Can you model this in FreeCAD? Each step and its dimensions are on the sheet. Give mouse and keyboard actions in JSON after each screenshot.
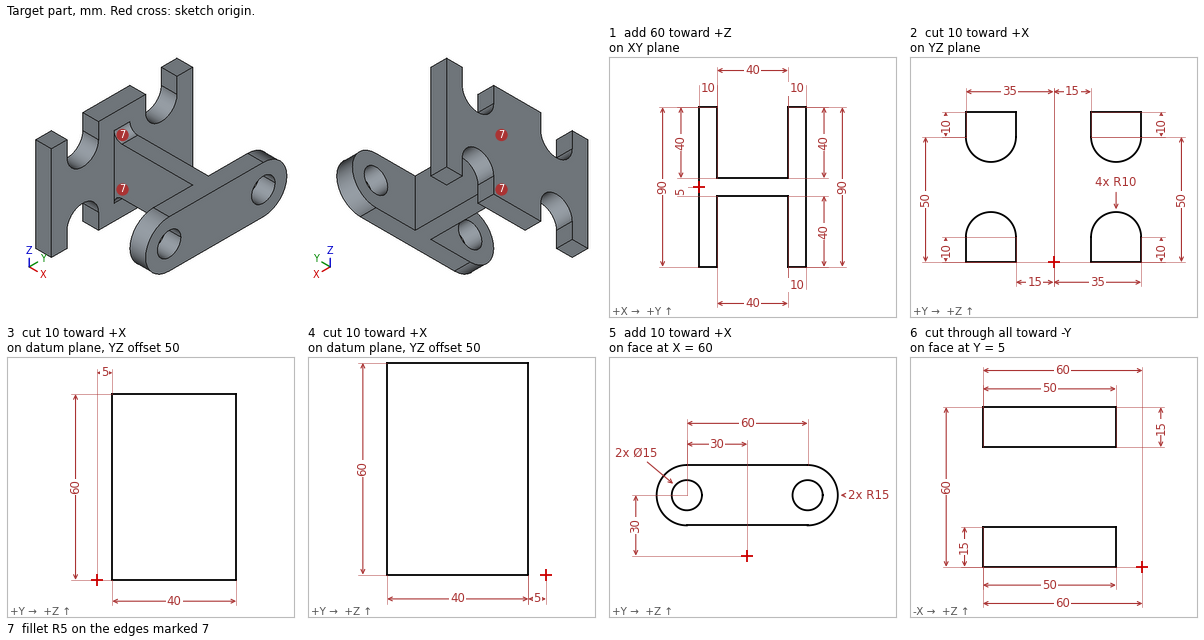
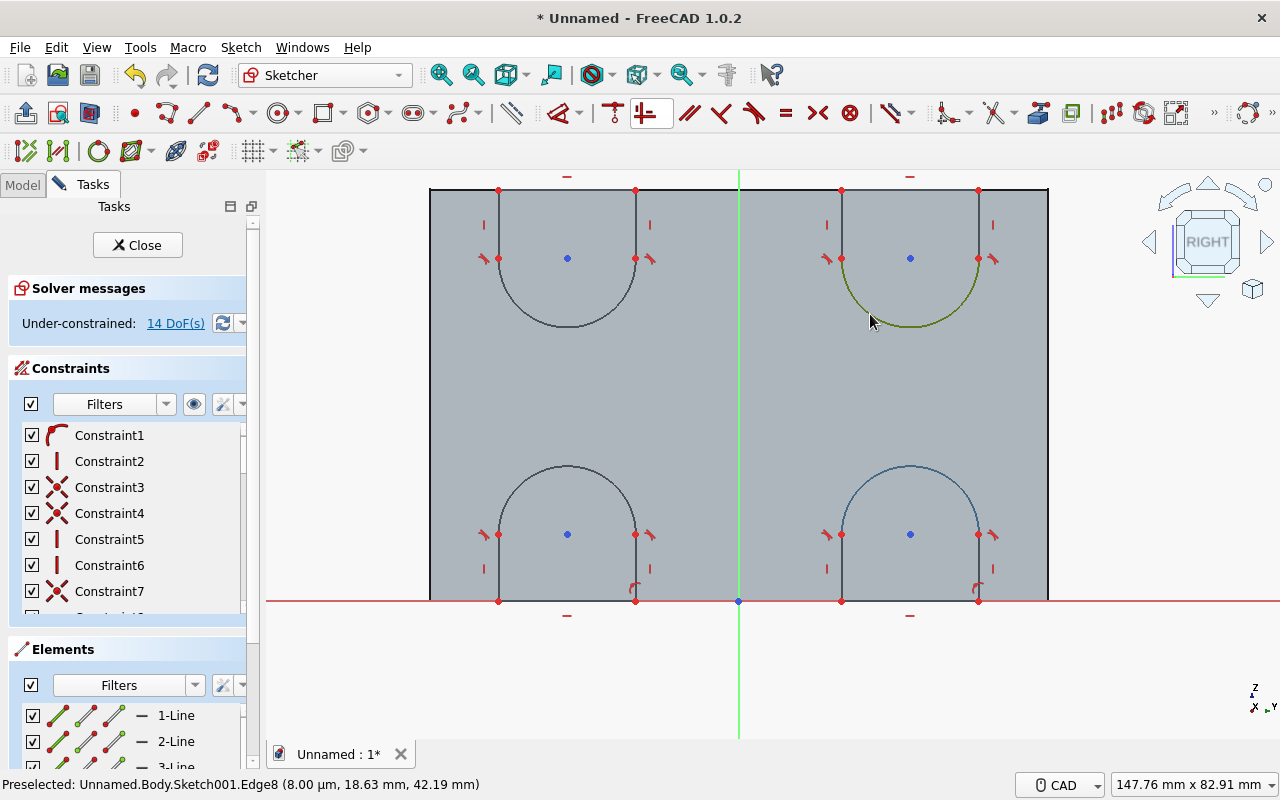
{"action": "left_click", "coordinate": [608, 479]}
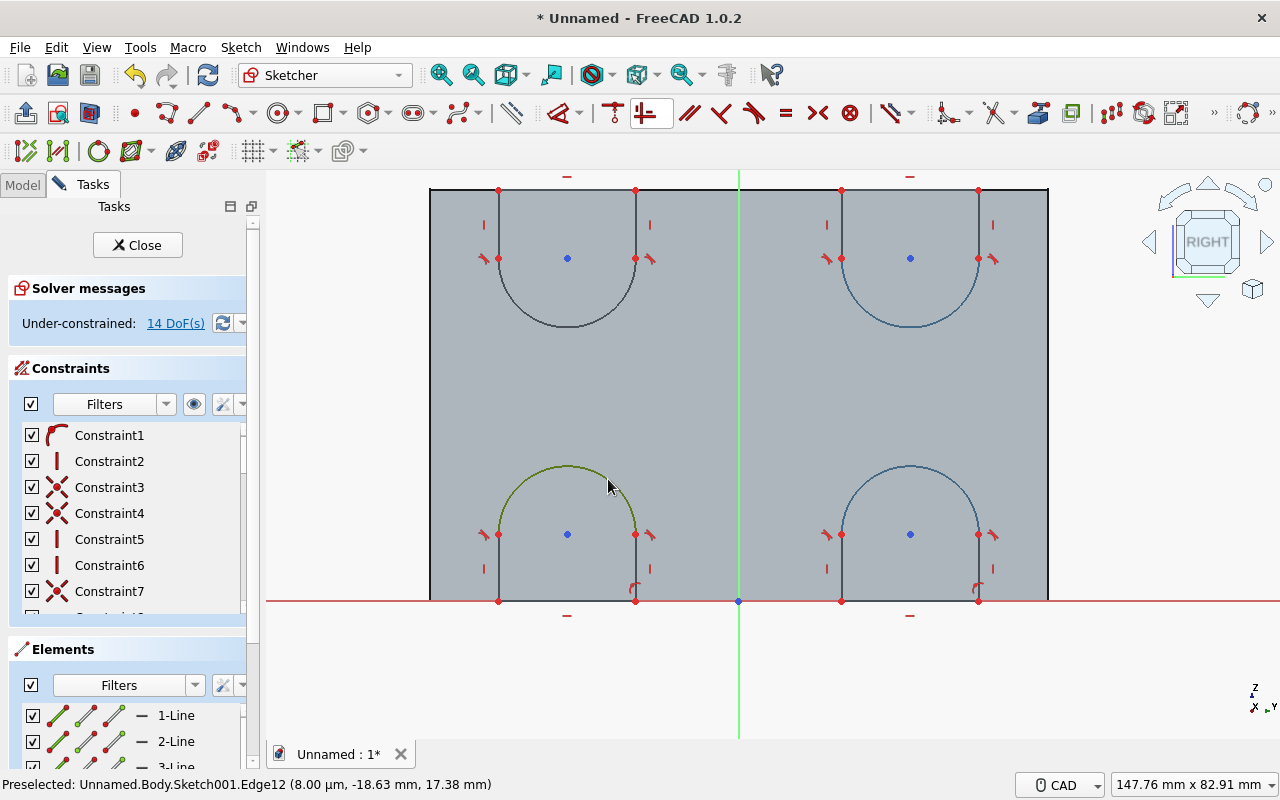
{"action": "left_click", "coordinate": [527, 314]}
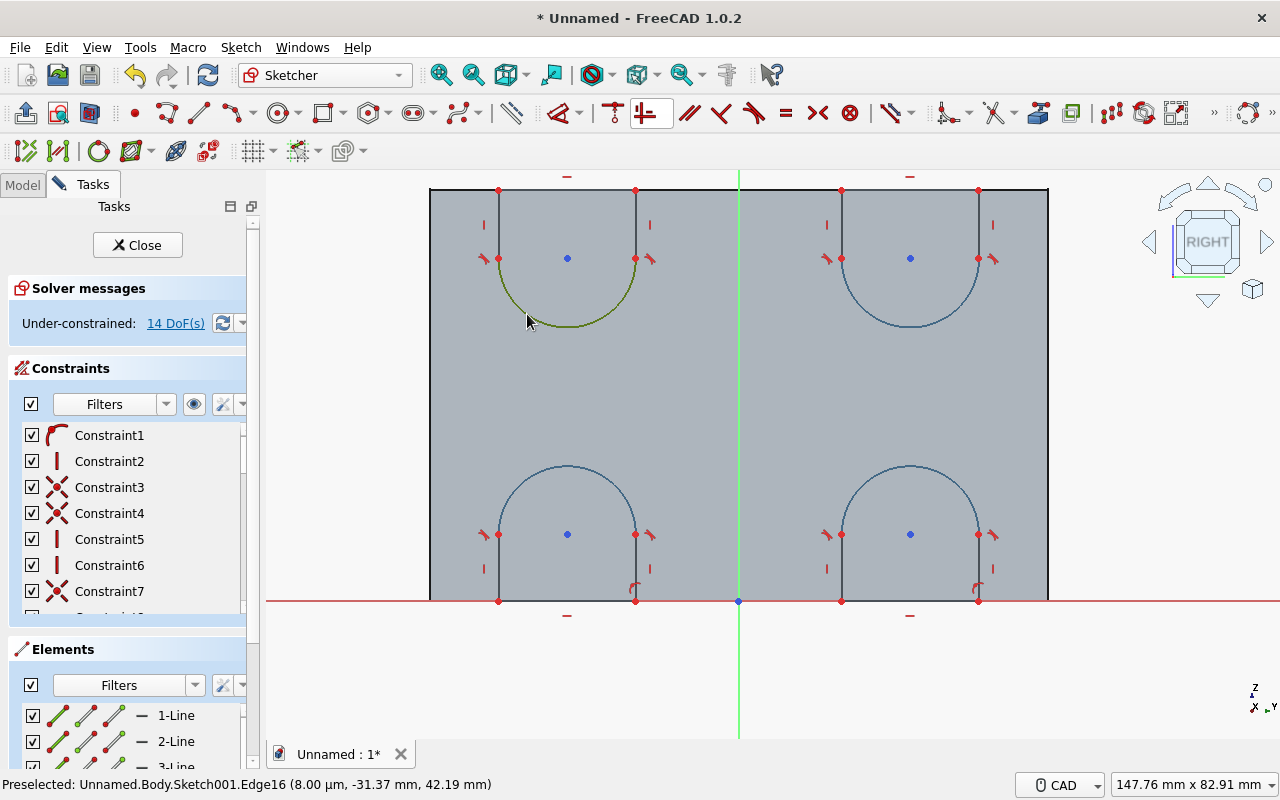
{"action": "left_click", "coordinate": [786, 114]}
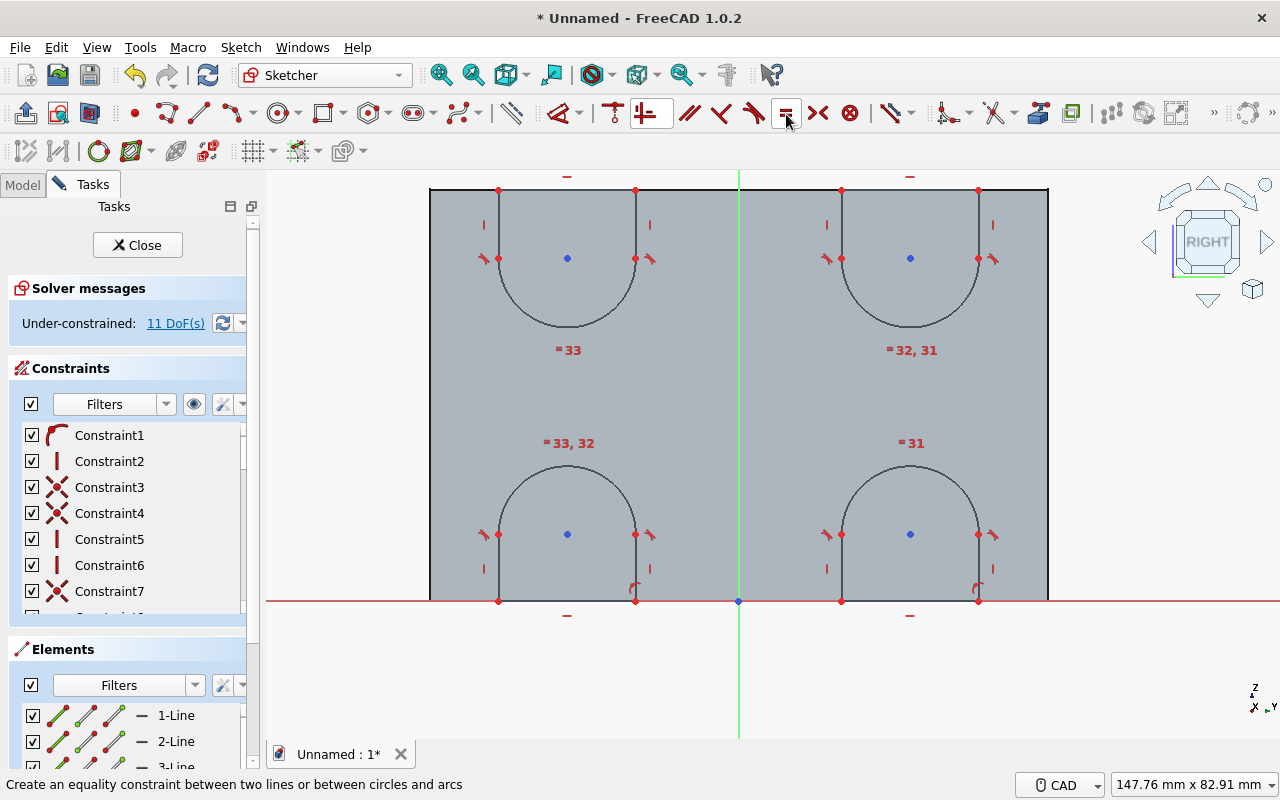
{"action": "left_click", "coordinate": [558, 114]}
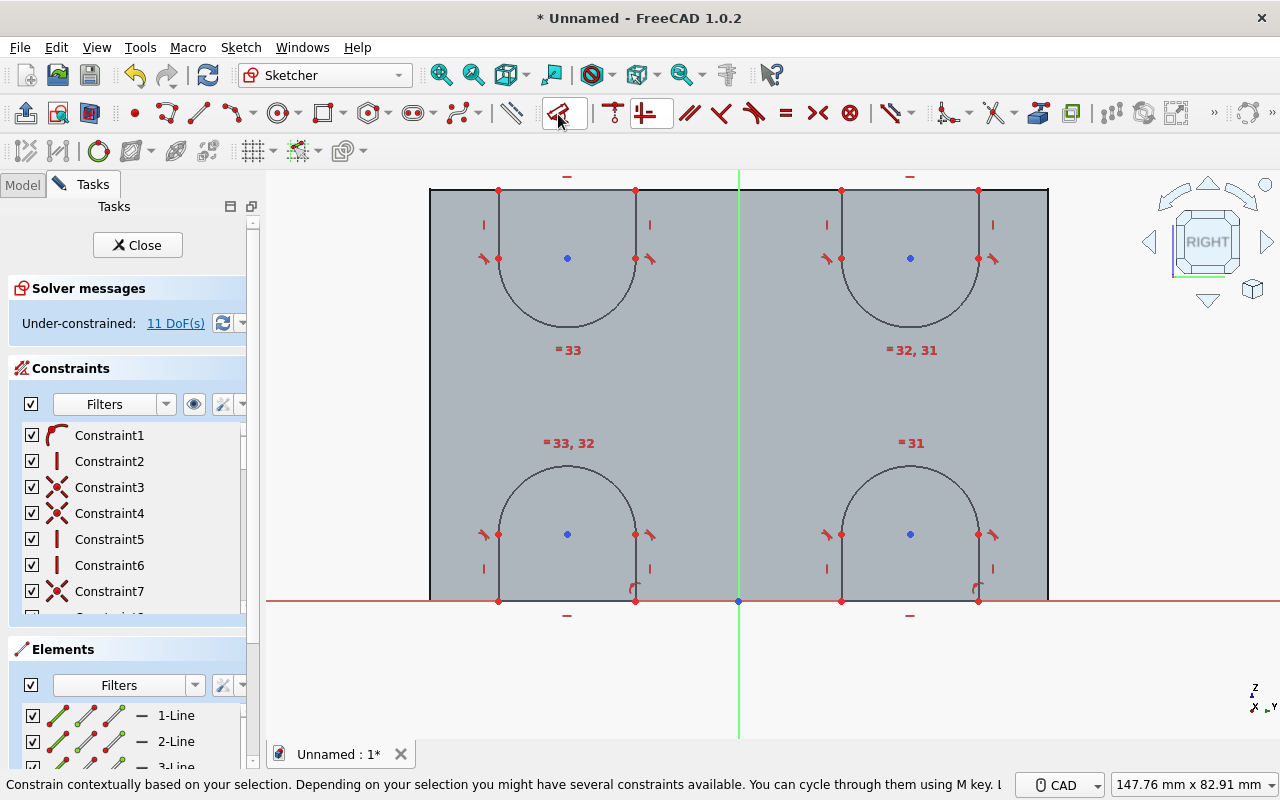
{"action": "left_click", "coordinate": [951, 479]}
{"action": "left_click", "coordinate": [970, 453]}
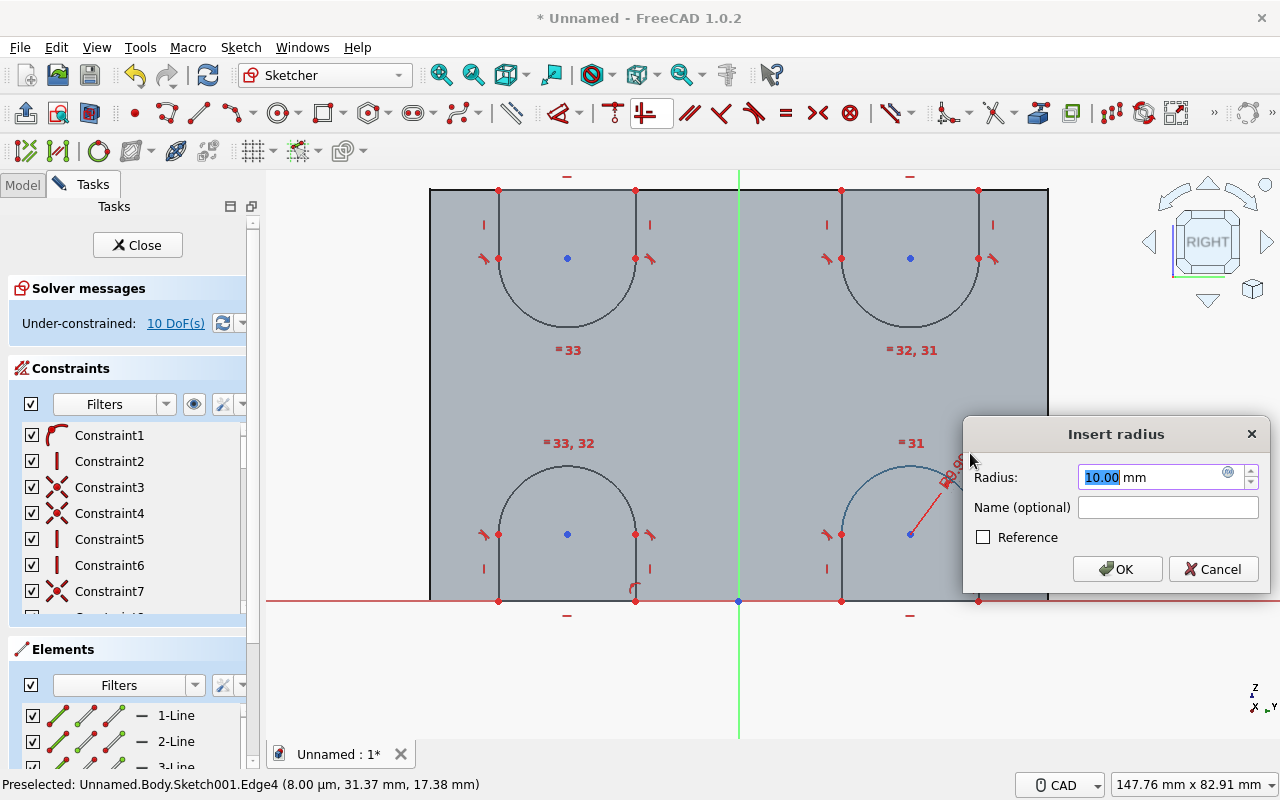
{"action": "type", "text": "10"}
{"action": "key", "text": "Return"}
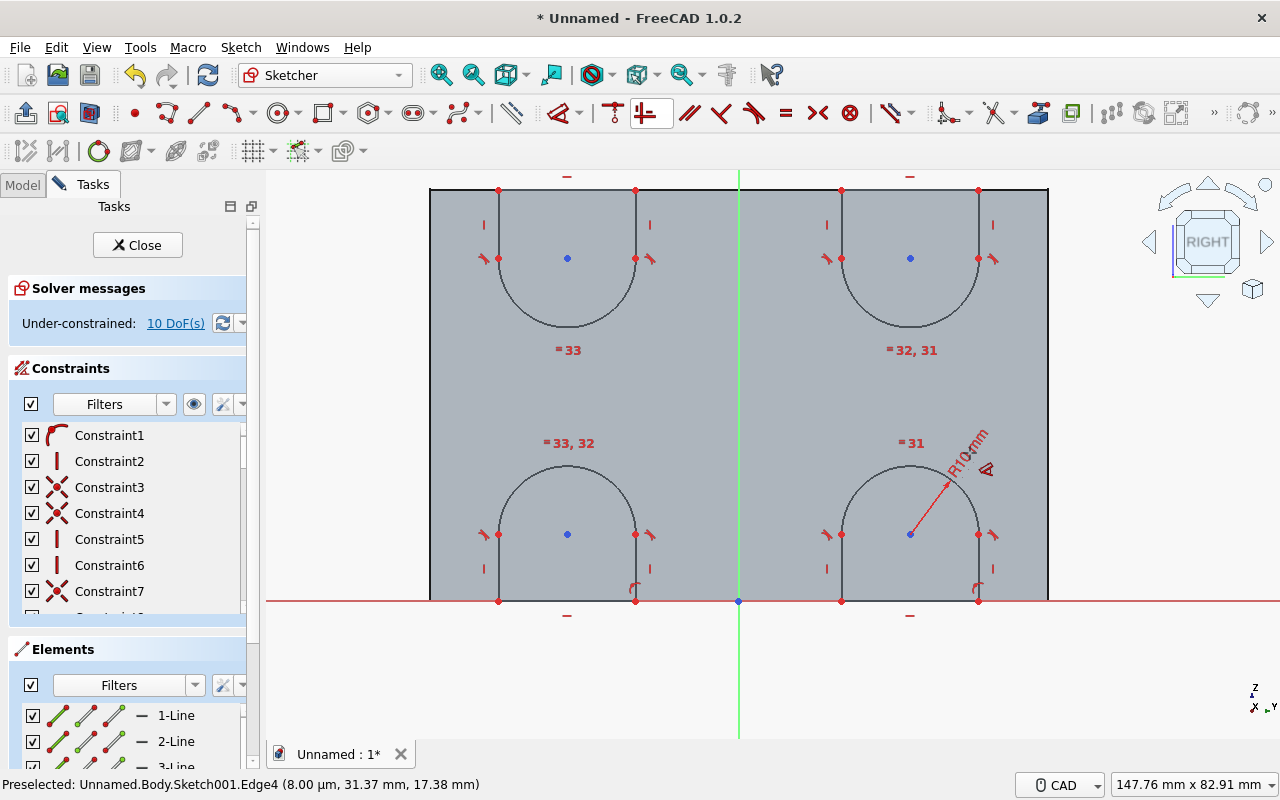
{"action": "left_click", "coordinate": [979, 555]}
{"action": "left_click", "coordinate": [1013, 568]}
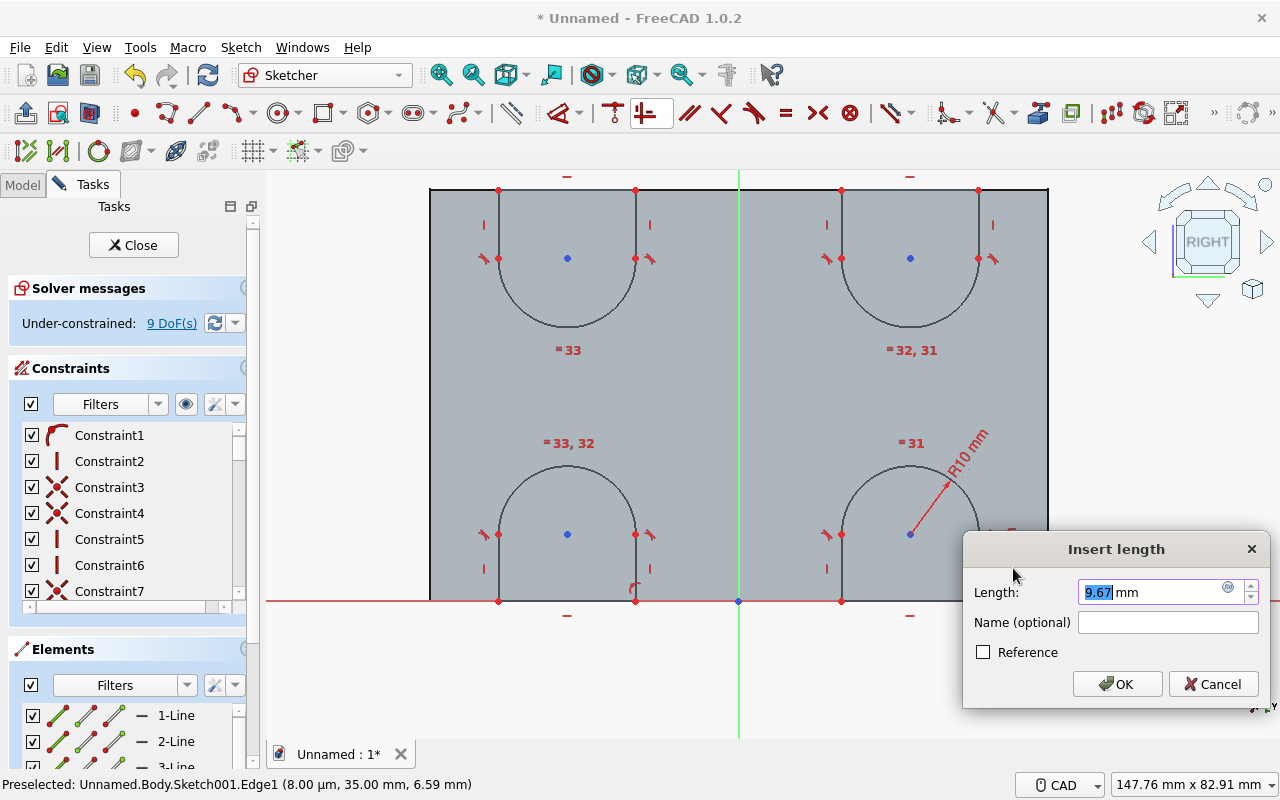
{"action": "type", "text": "10"}
{"action": "key", "text": "Return"}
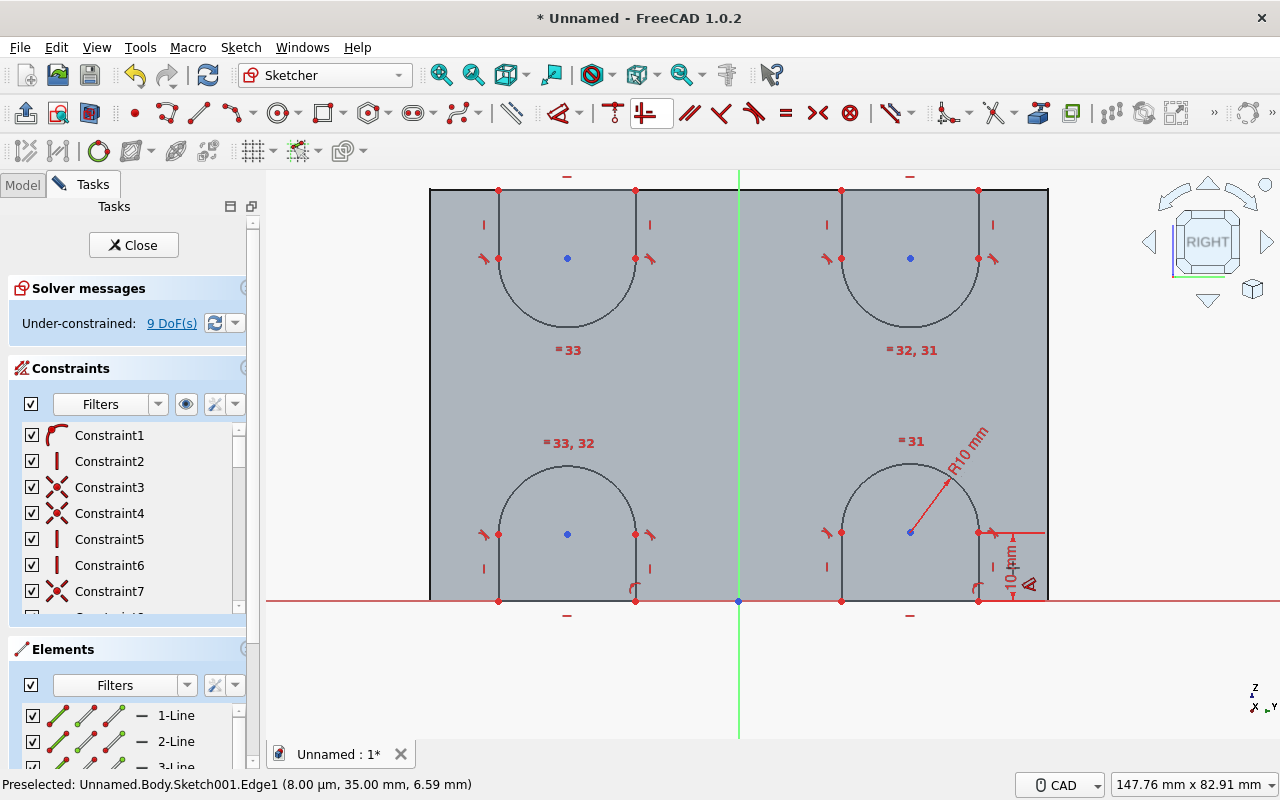
{"action": "left_click", "coordinate": [842, 238]}
{"action": "left_click", "coordinate": [876, 228]}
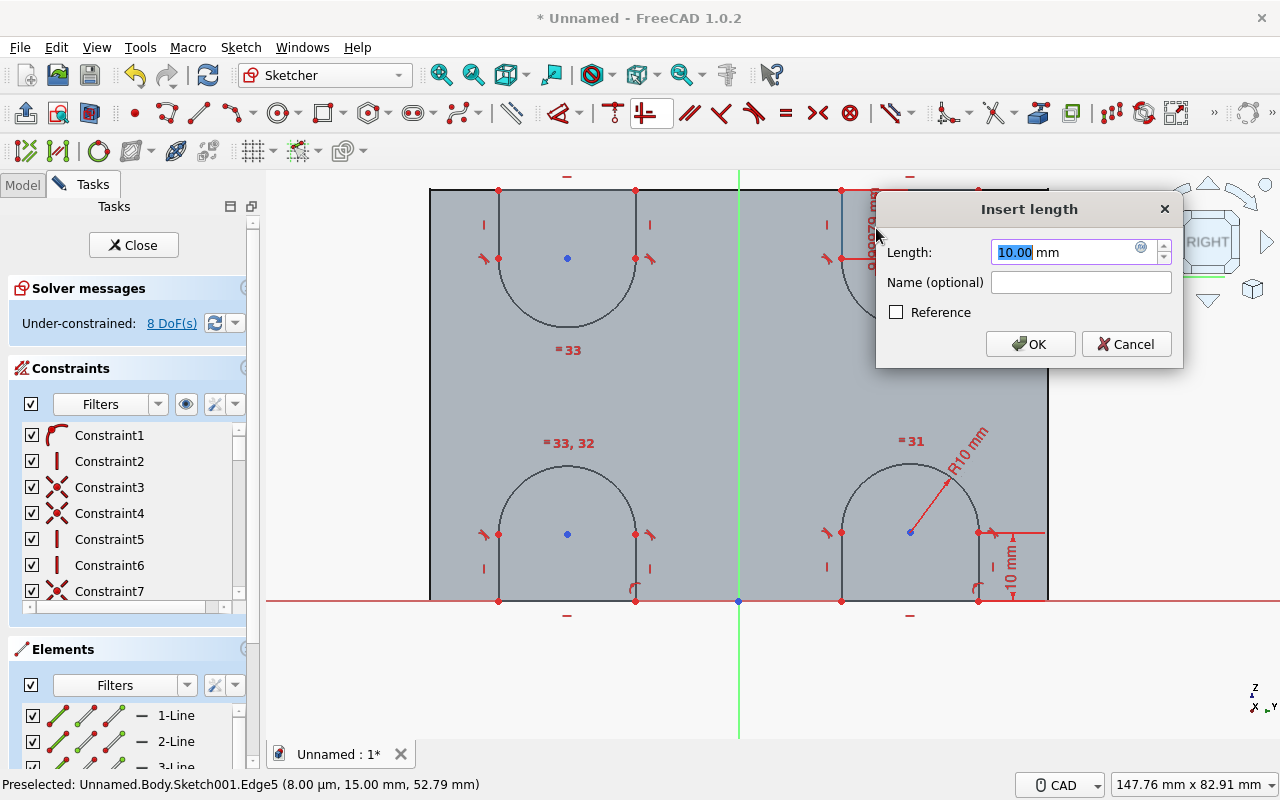
{"action": "type", "text": "10"}
{"action": "key", "text": "Return"}